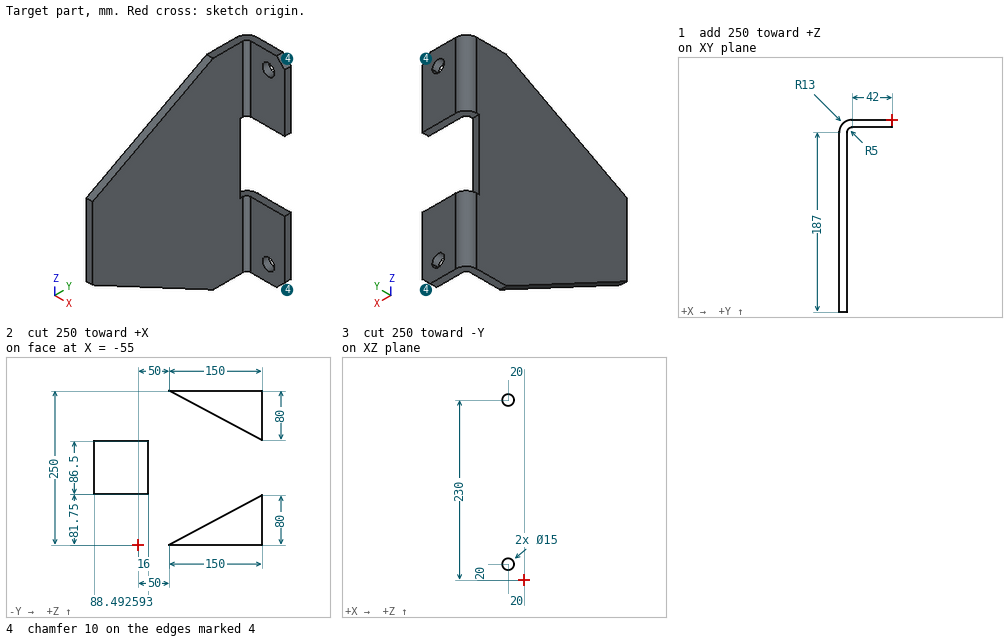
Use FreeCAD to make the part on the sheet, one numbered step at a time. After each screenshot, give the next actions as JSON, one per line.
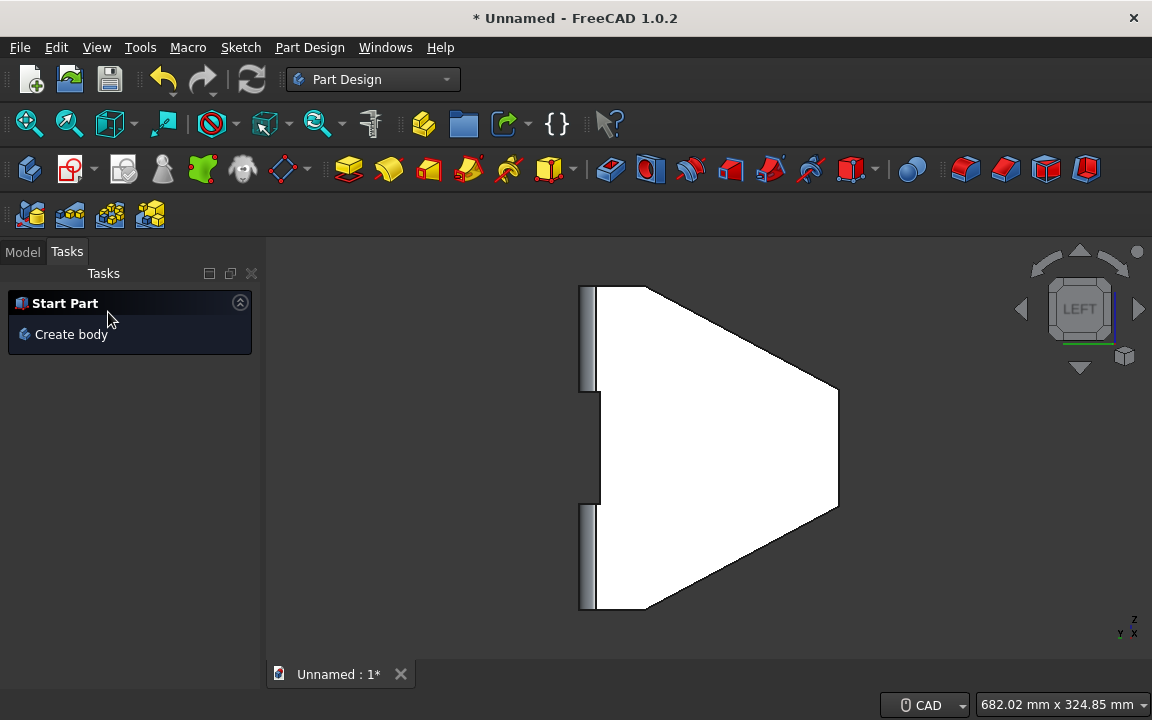
{"action": "scroll", "coordinate": [584, 285], "scroll_direction": "up", "scroll_amount": 7}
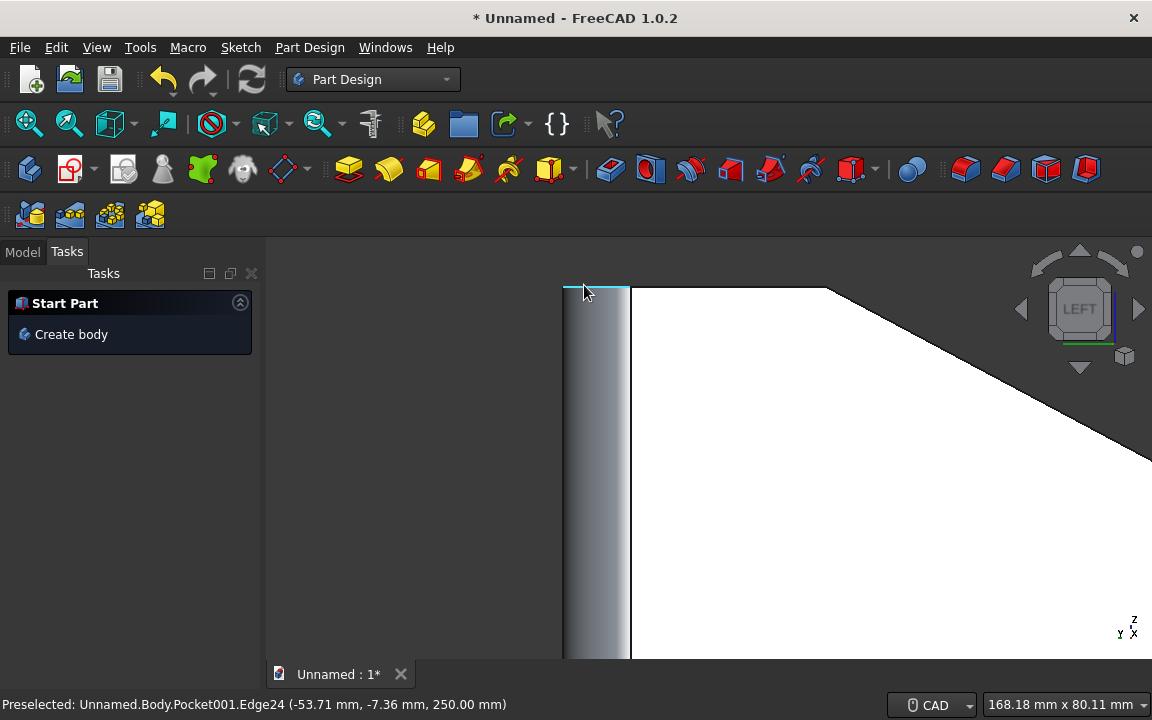
{"action": "left_click", "coordinate": [30, 124]}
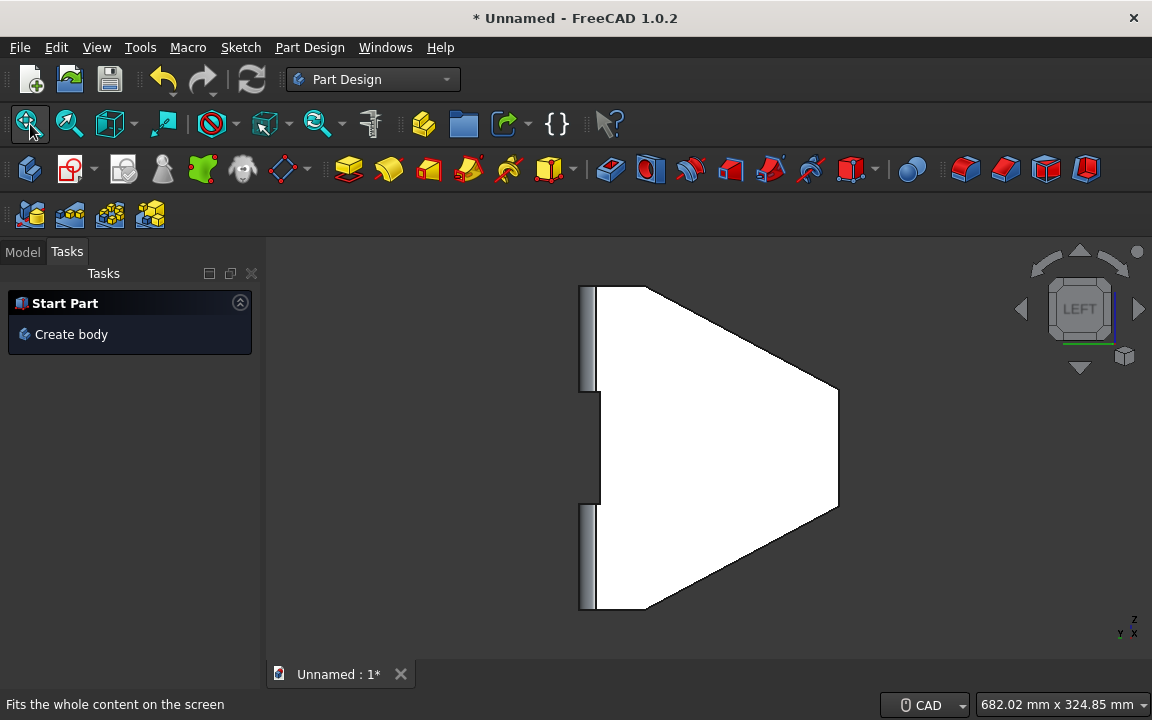
{"action": "key", "text": "0"}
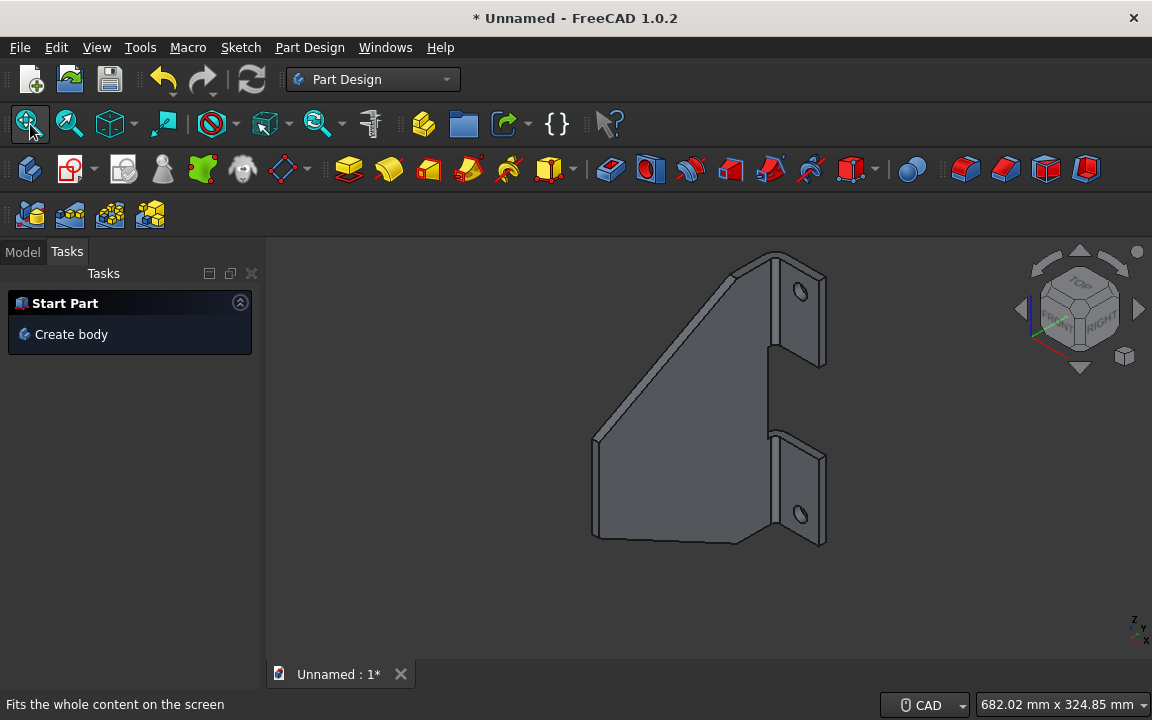
{"action": "left_click", "coordinate": [825, 277]}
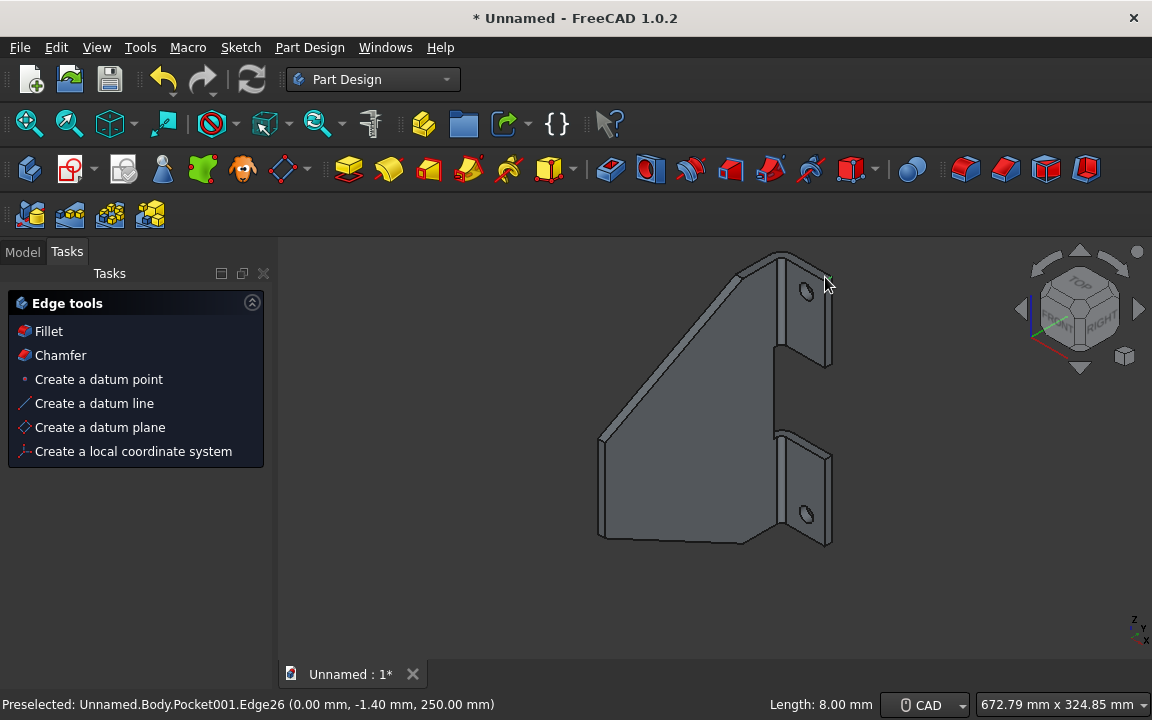
{"action": "scroll", "coordinate": [828, 543], "scroll_direction": "up", "scroll_amount": 7}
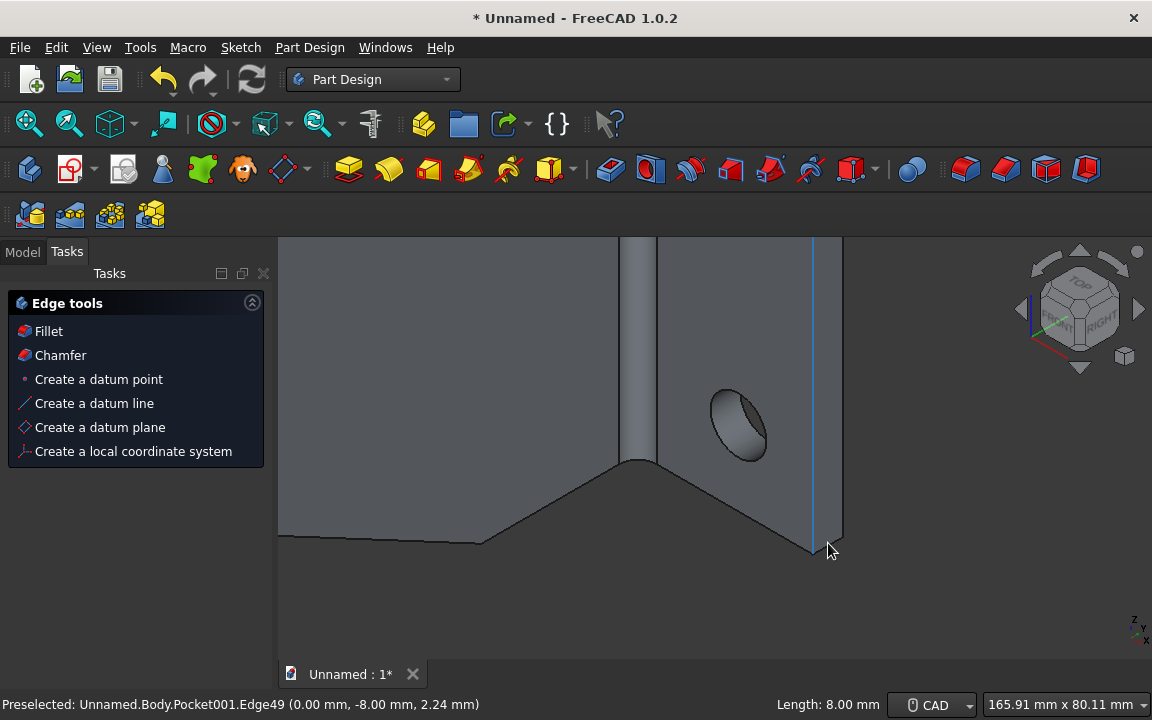
{"action": "left_click", "coordinate": [30, 124]}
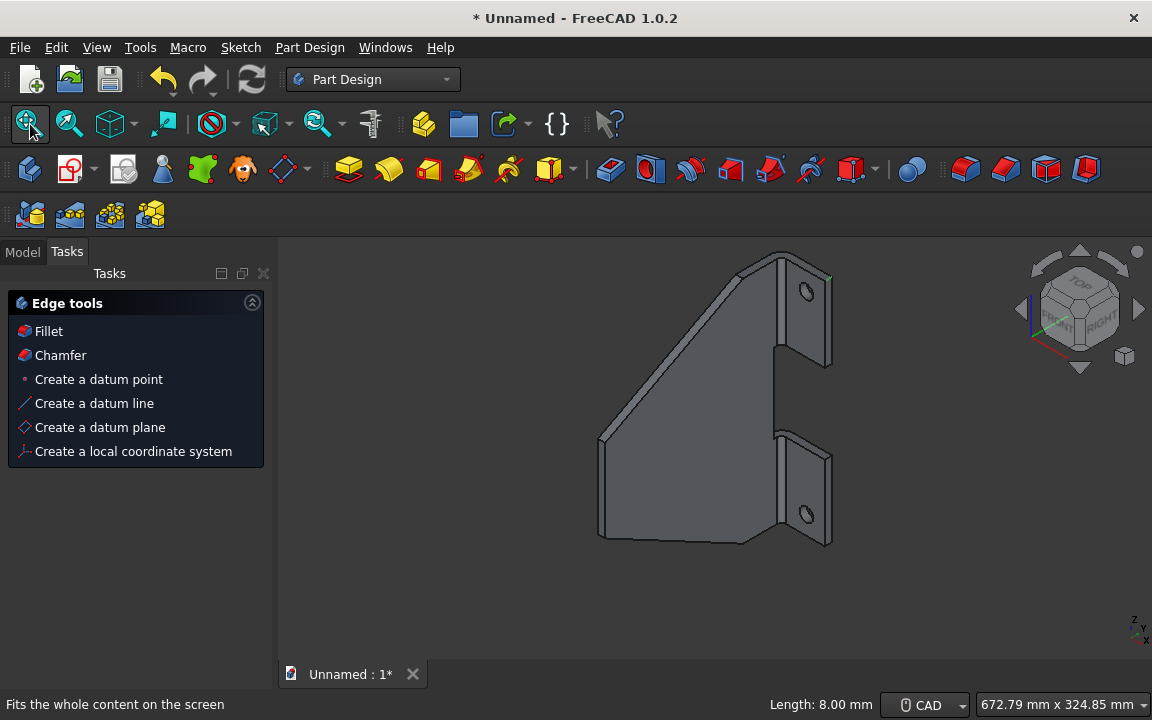
{"action": "key", "text": "2"}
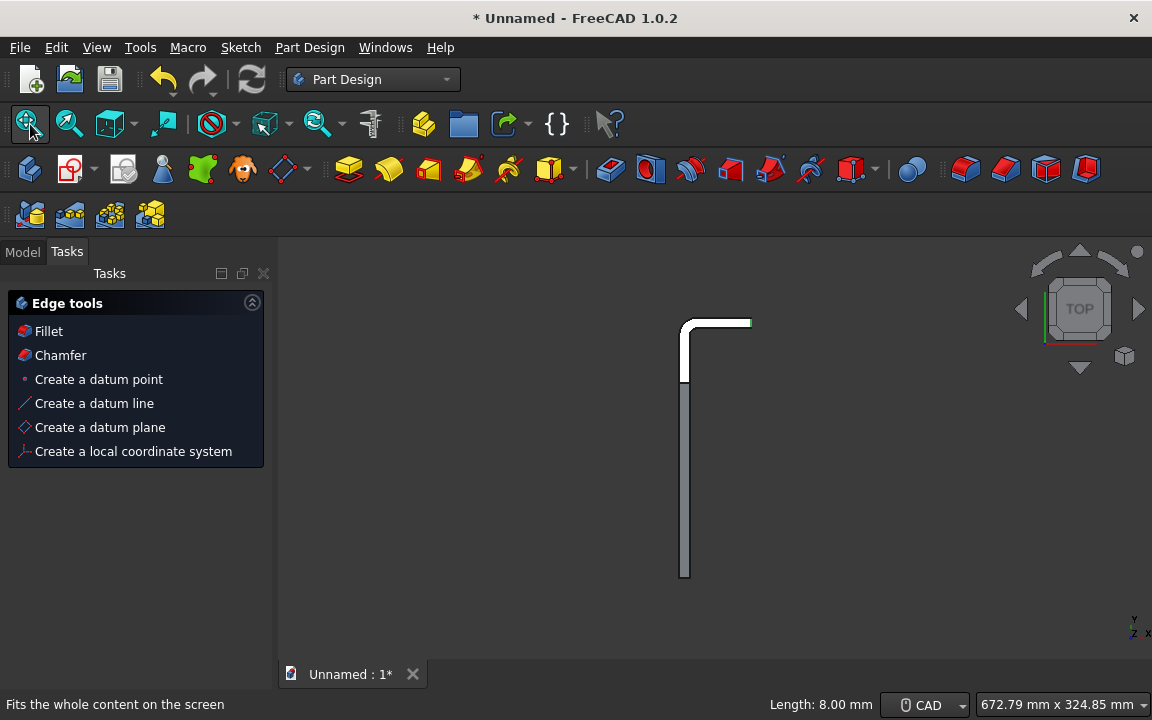
{"action": "scroll", "coordinate": [751, 322], "scroll_direction": "up", "scroll_amount": 7}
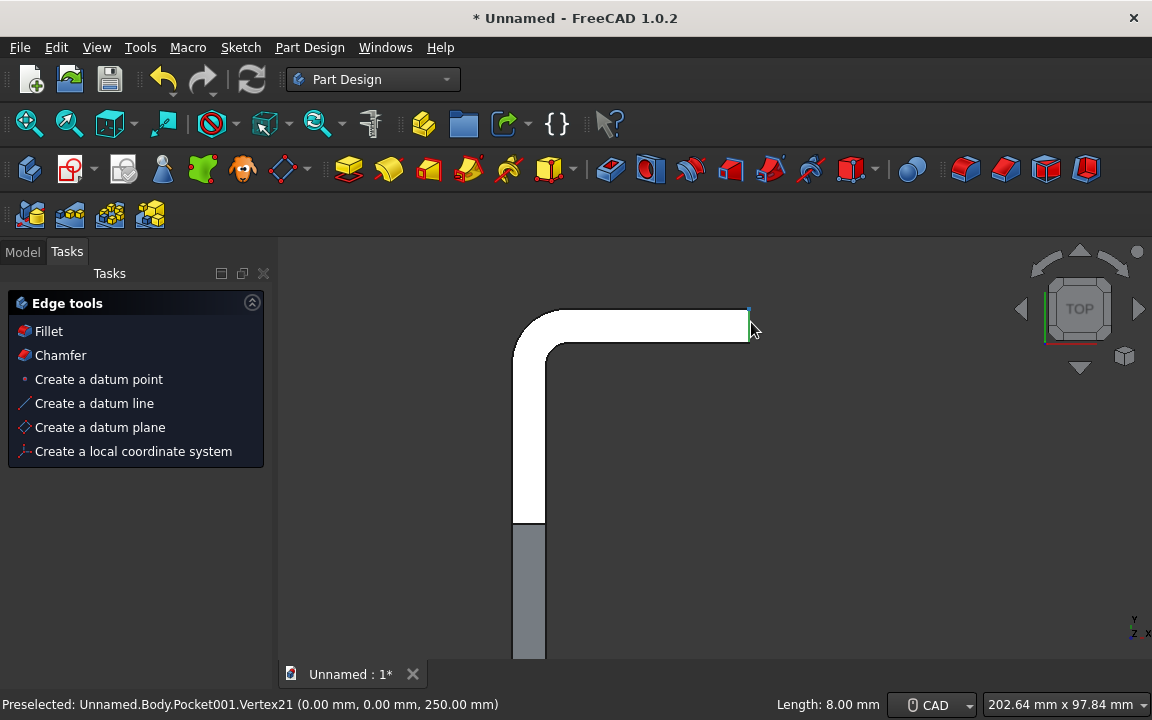
{"action": "key", "text": "v f"}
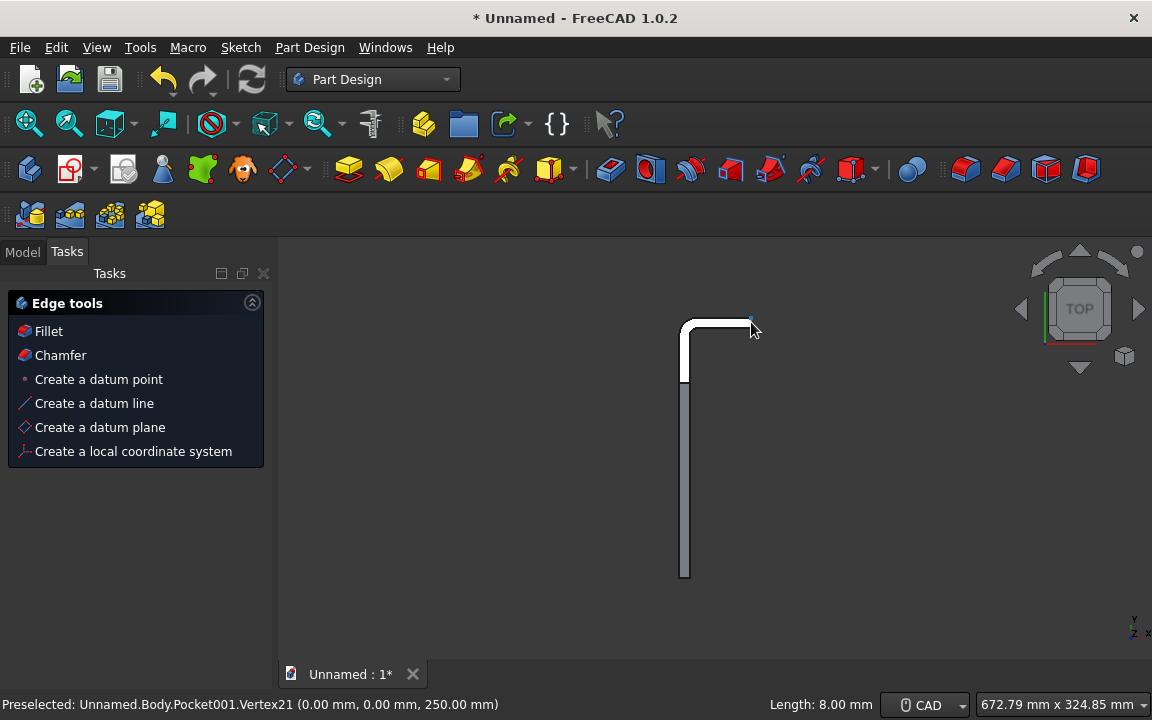
{"action": "key", "text": "1"}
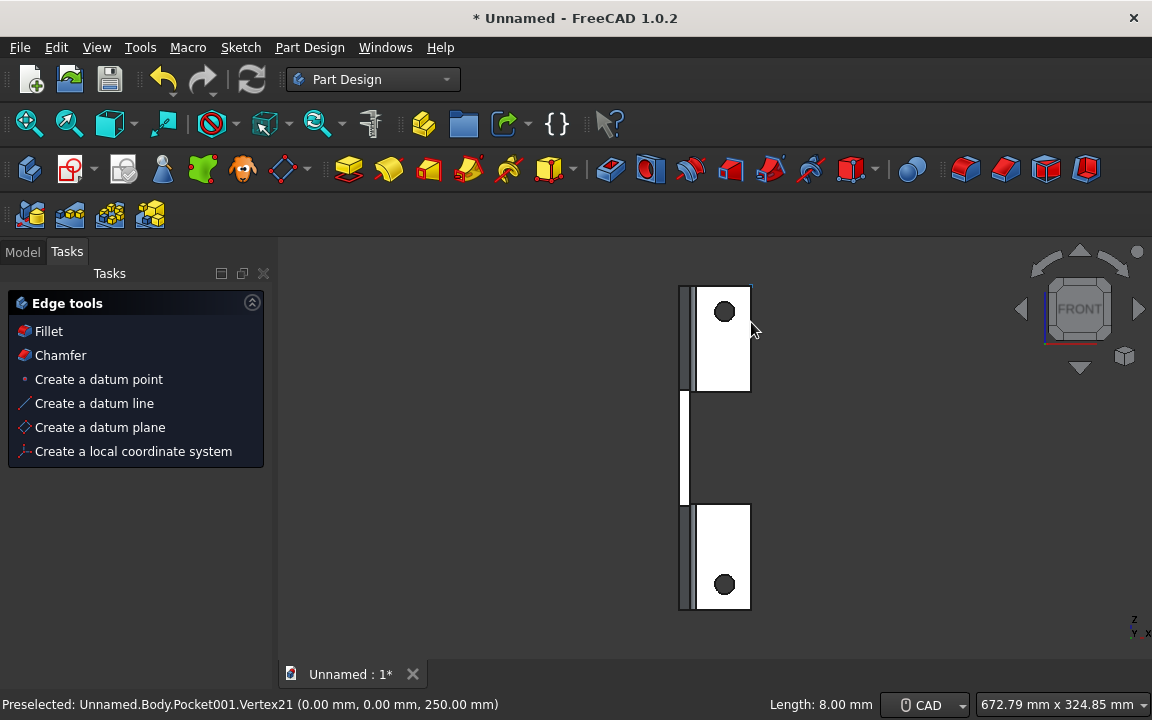
{"action": "scroll", "coordinate": [751, 609], "scroll_direction": "up", "scroll_amount": 7}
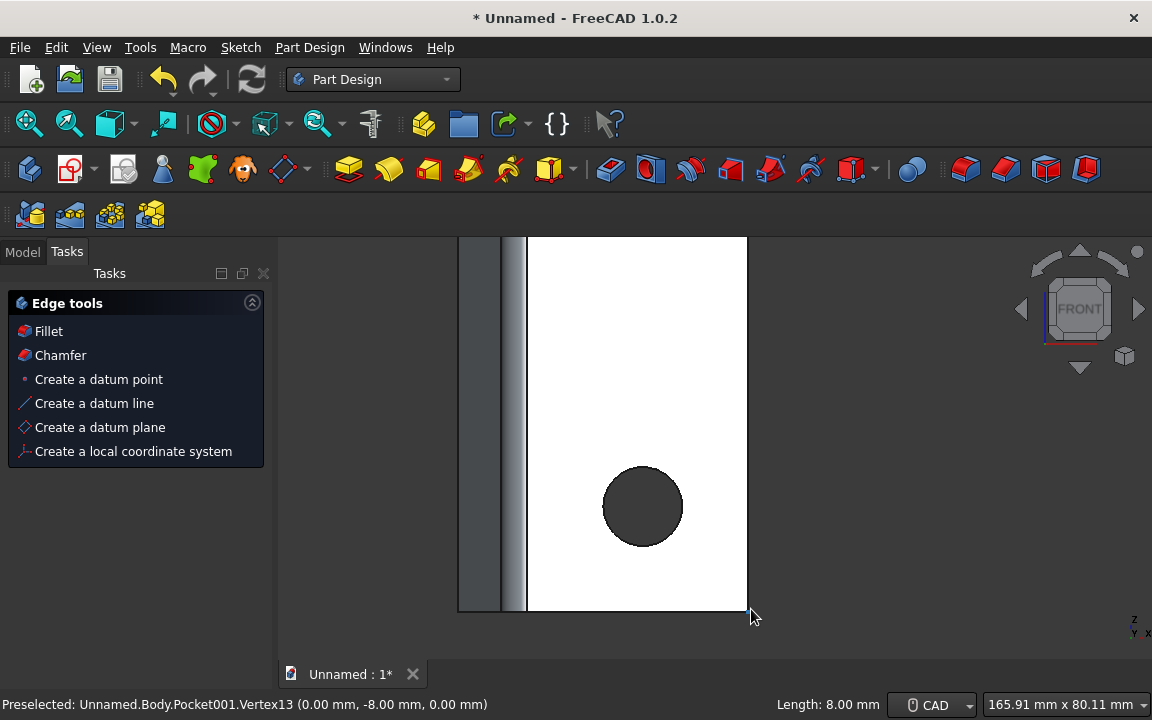
{"action": "left_click", "coordinate": [30, 124]}